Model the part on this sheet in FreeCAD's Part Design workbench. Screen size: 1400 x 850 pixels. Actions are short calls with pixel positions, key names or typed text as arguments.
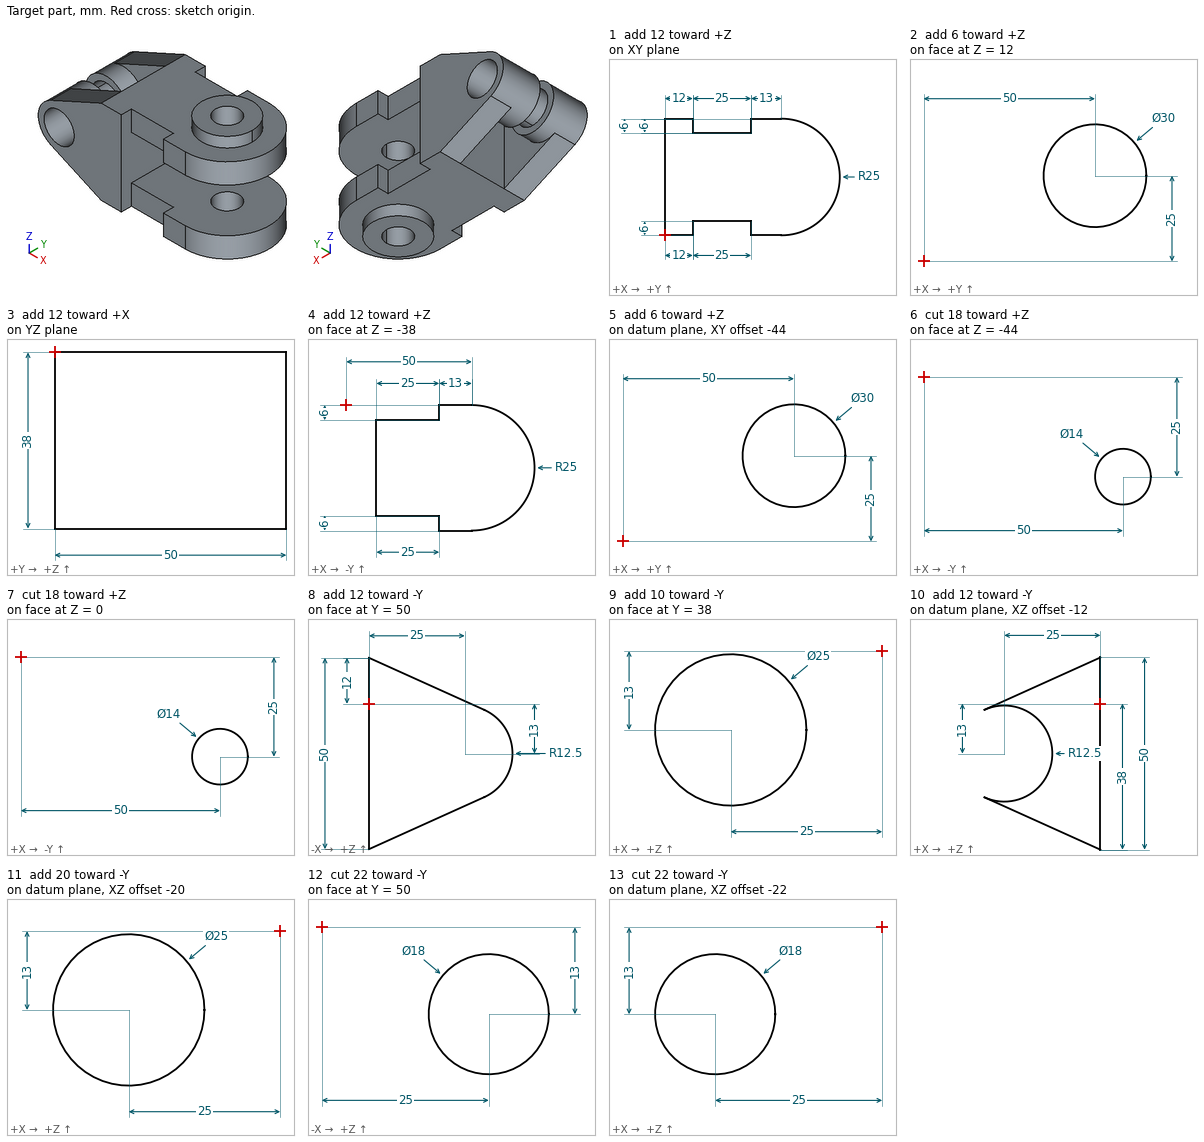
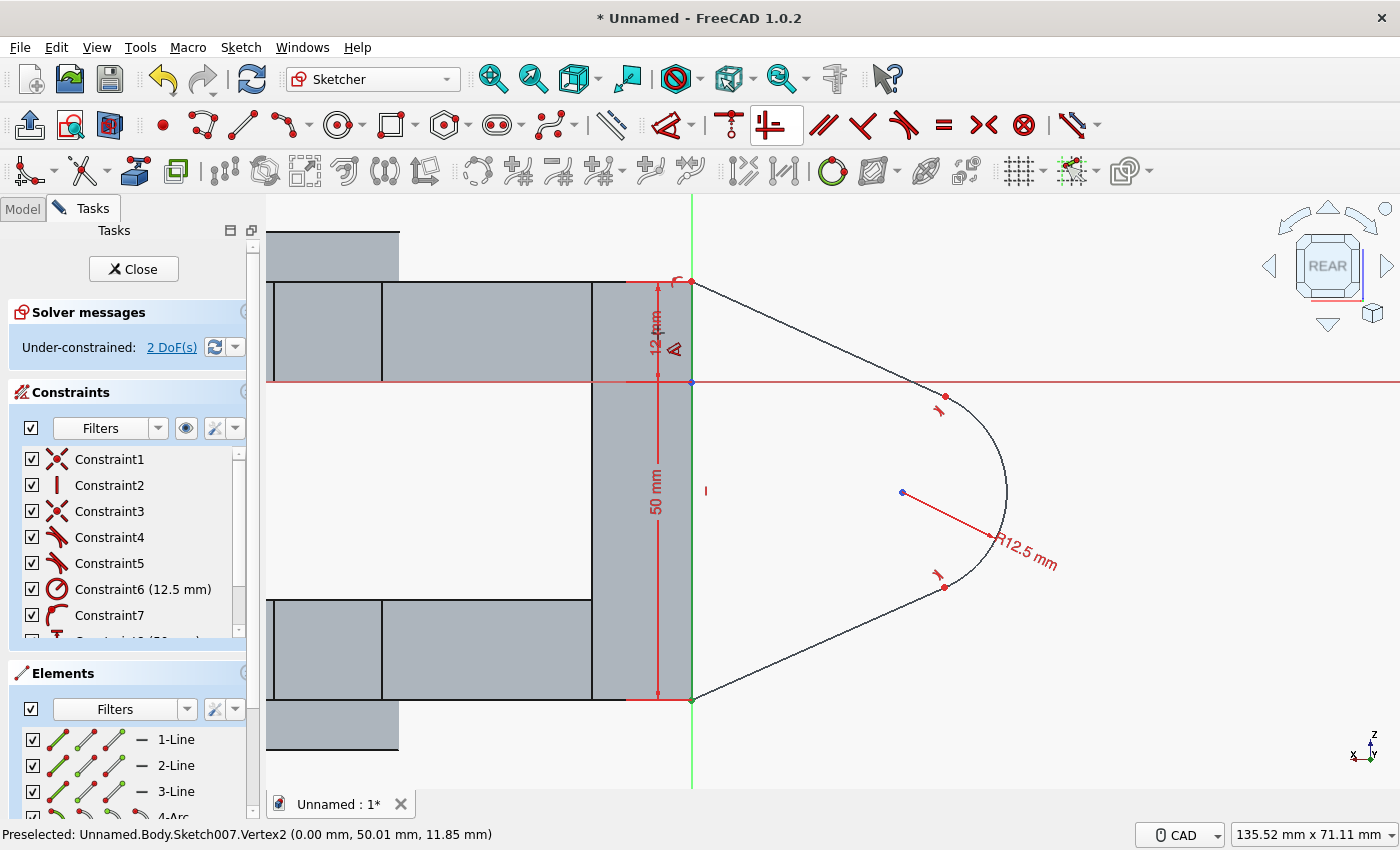
click(902, 492)
click(797, 348)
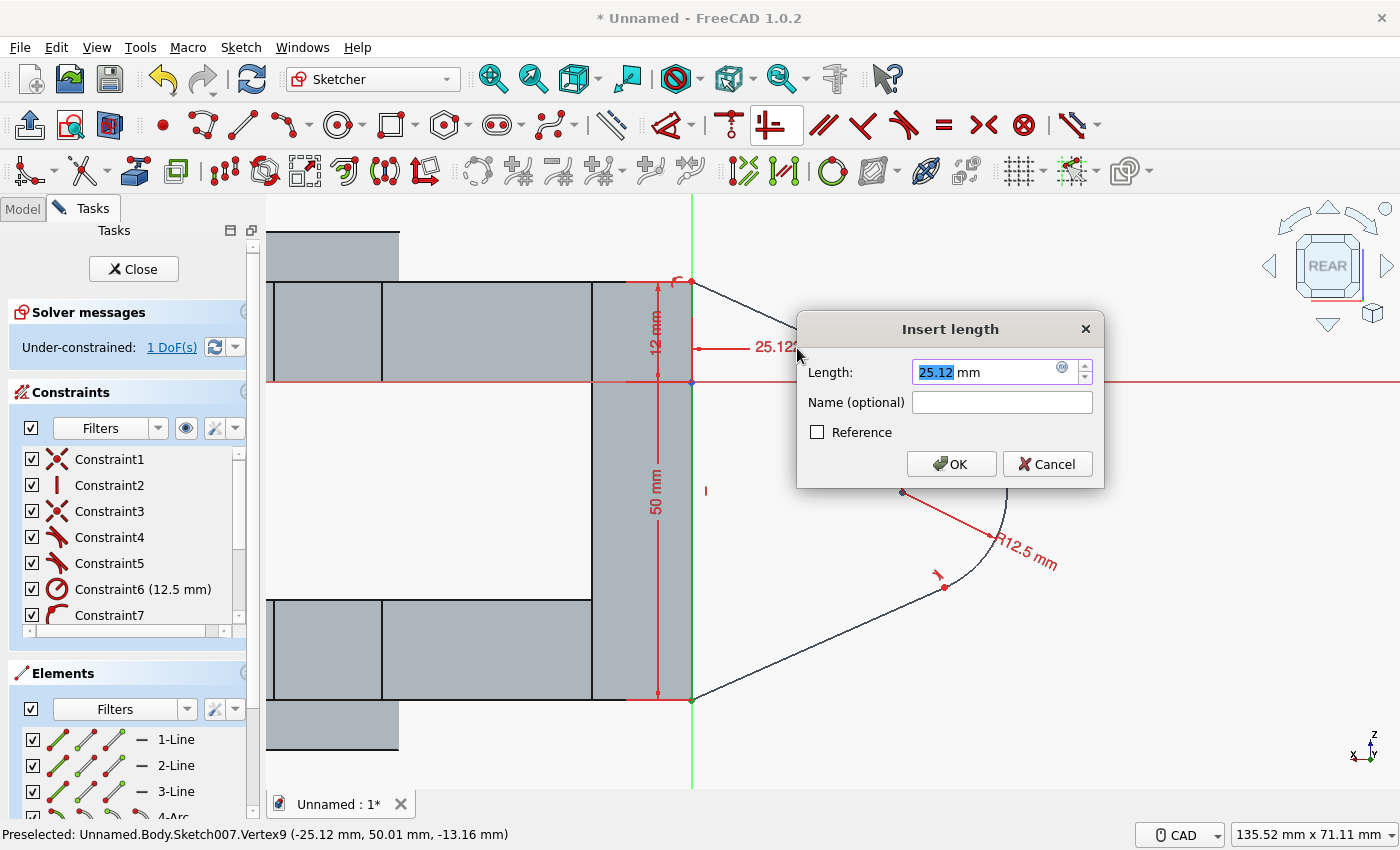
text(25)
key(Return)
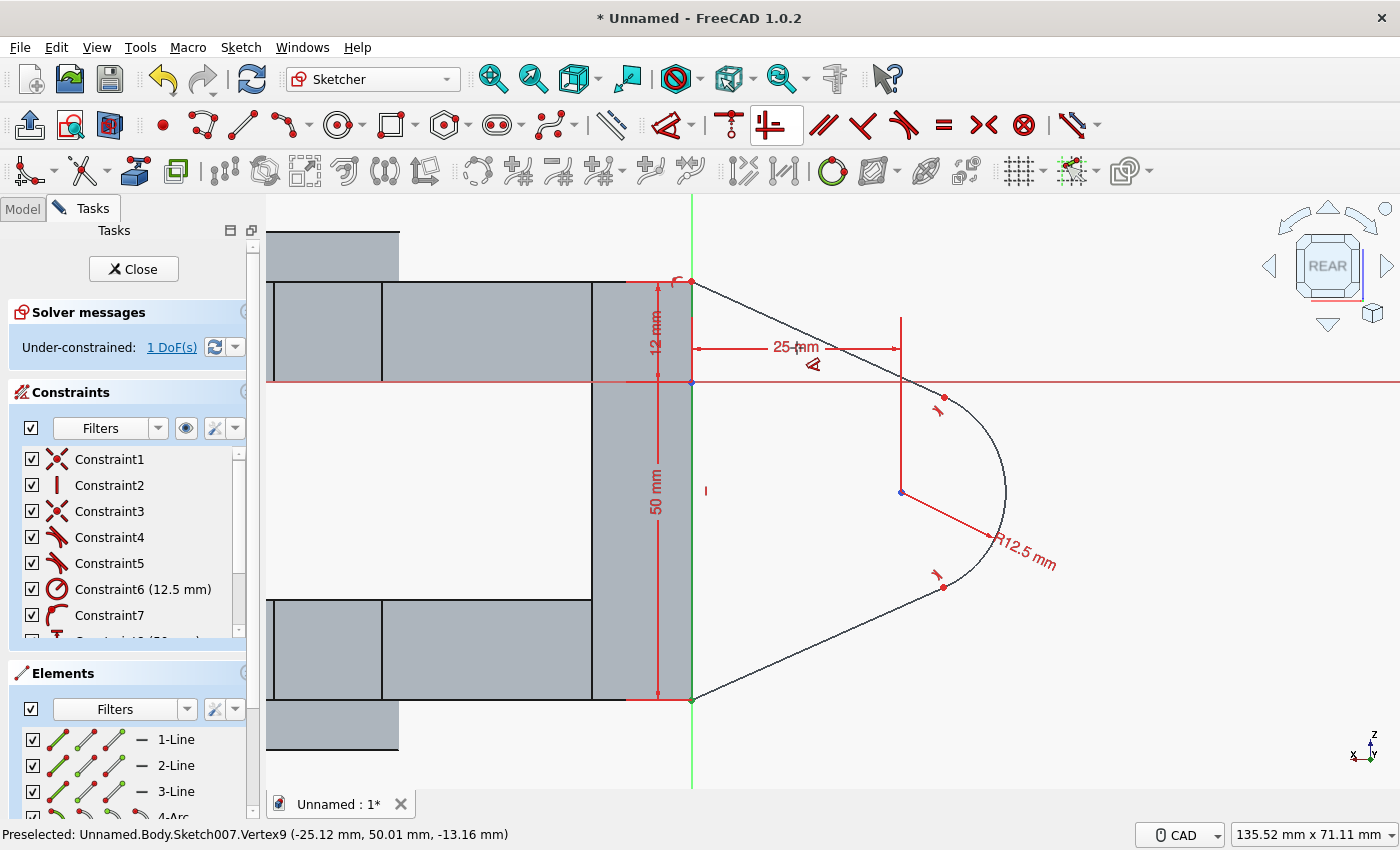
click(901, 492)
click(658, 437)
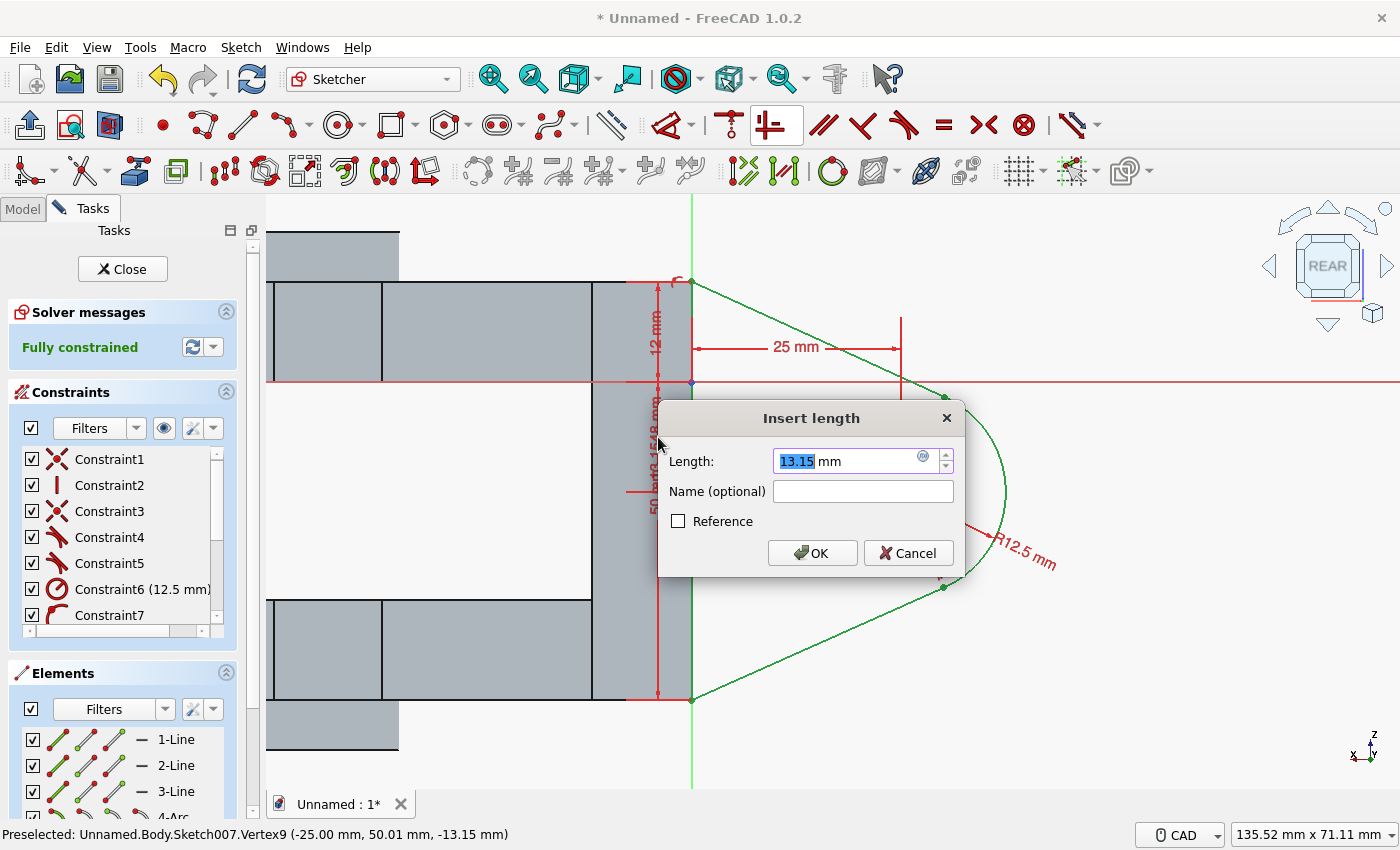
text(13)
key(Return)
key(Escape)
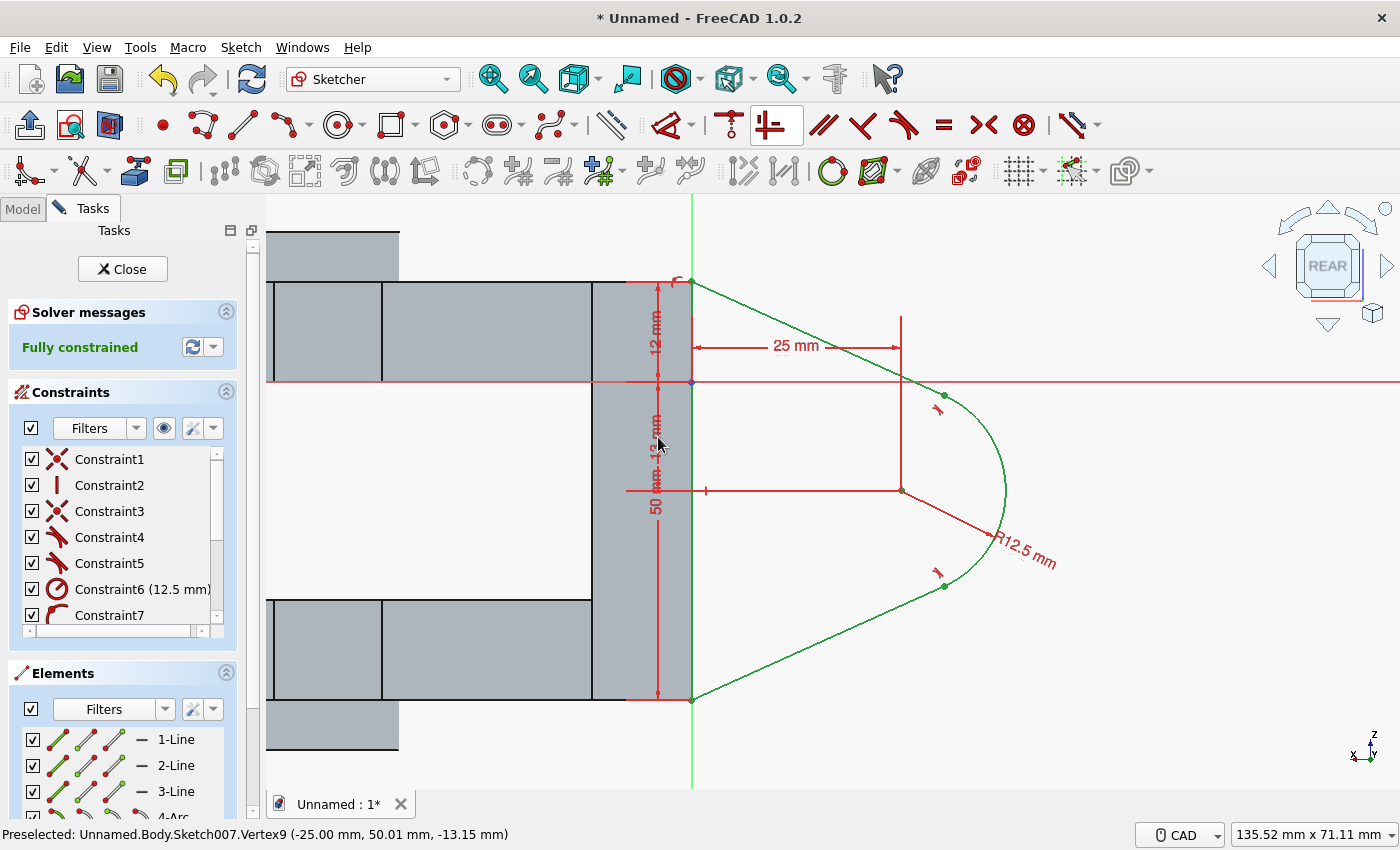
click(123, 269)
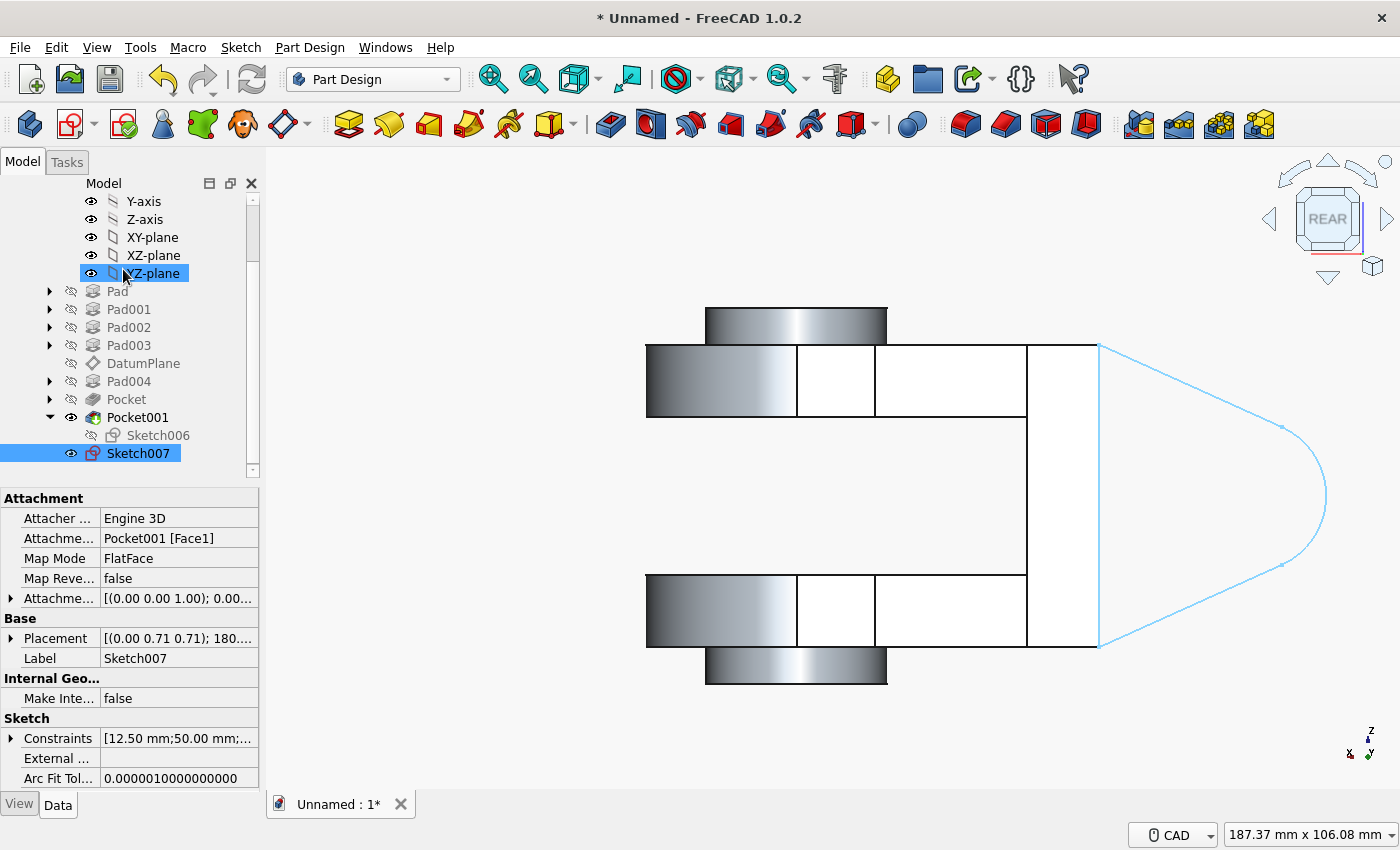
click(350, 124)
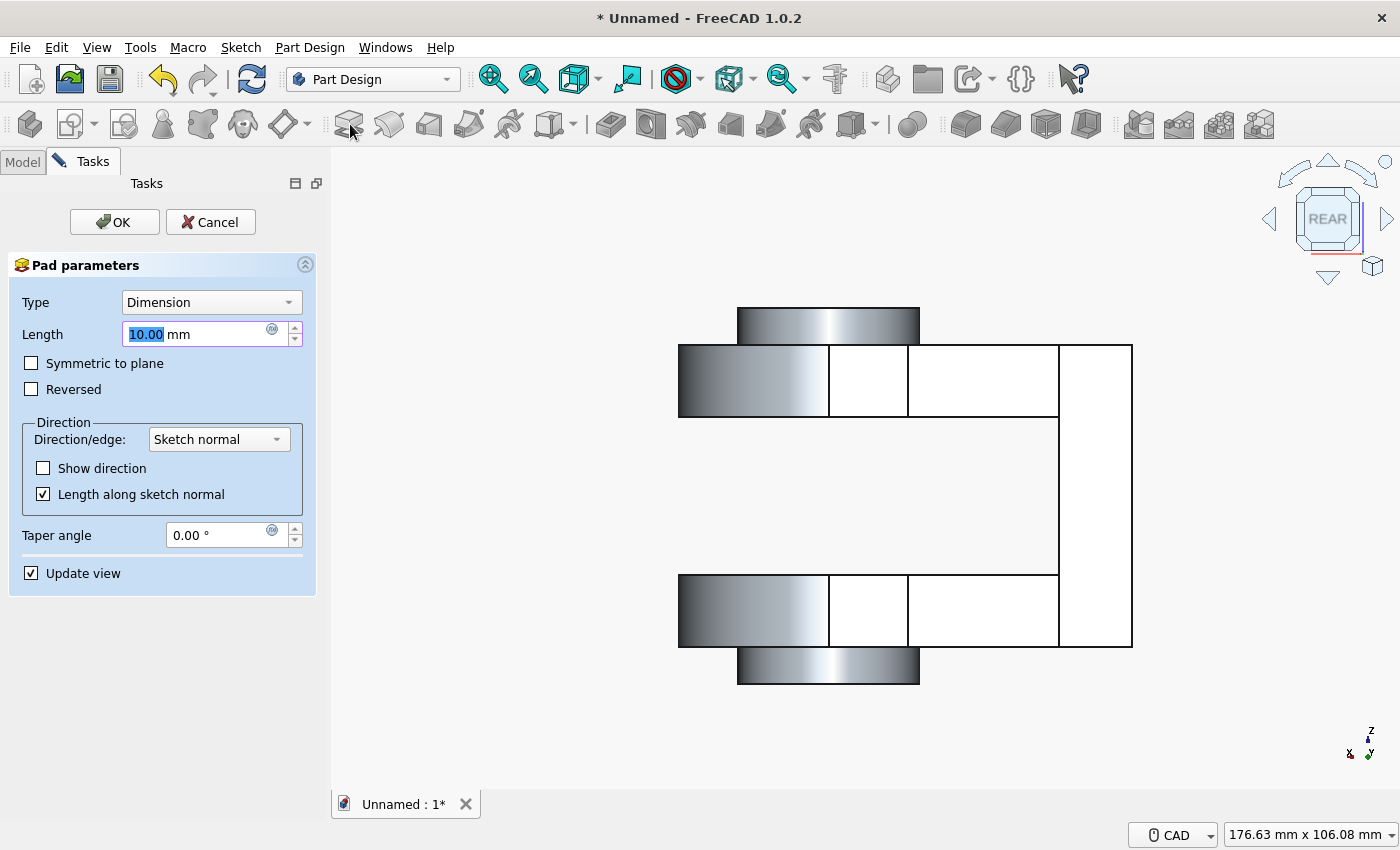
text(12)
key(Tab)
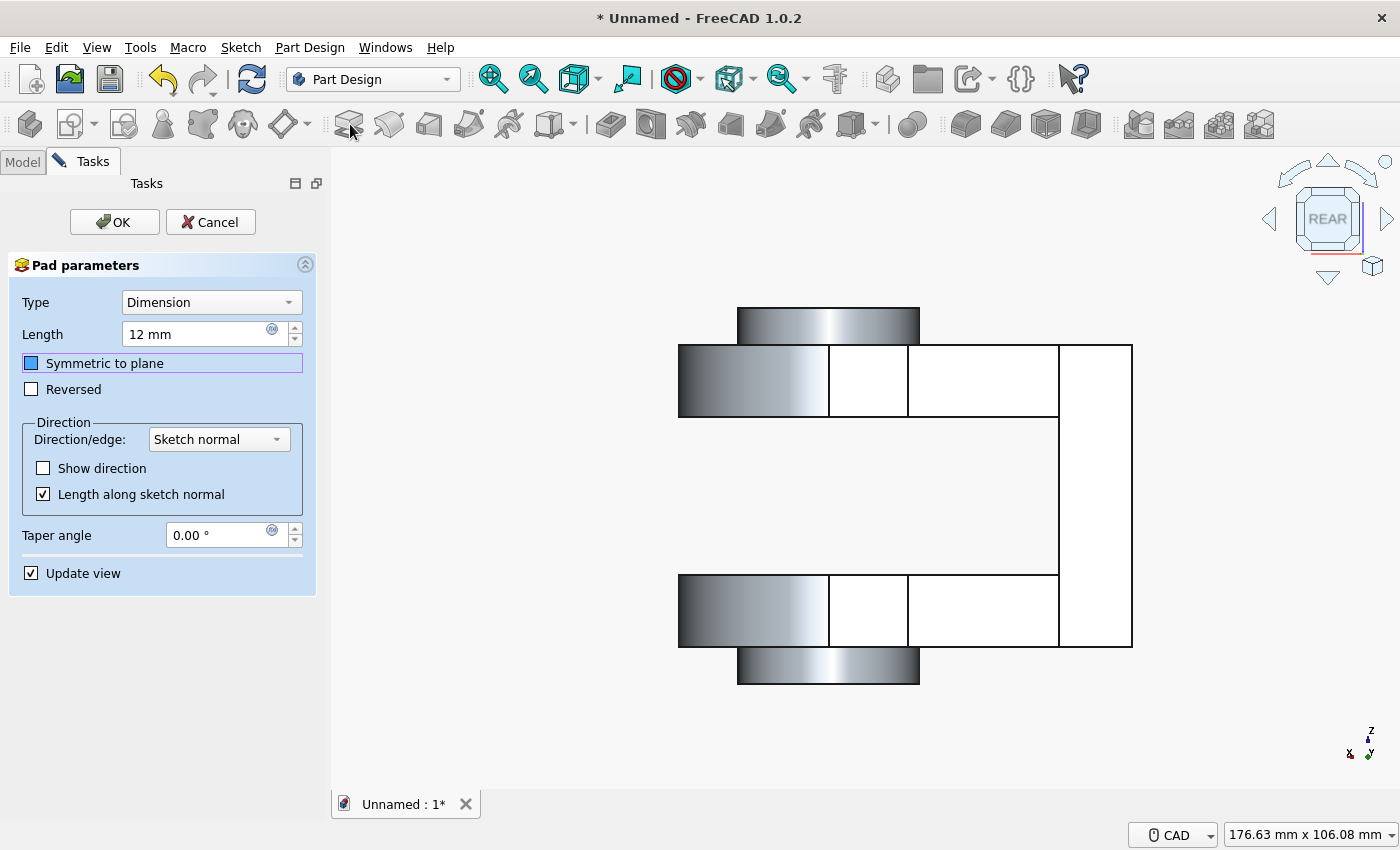
click(30, 389)